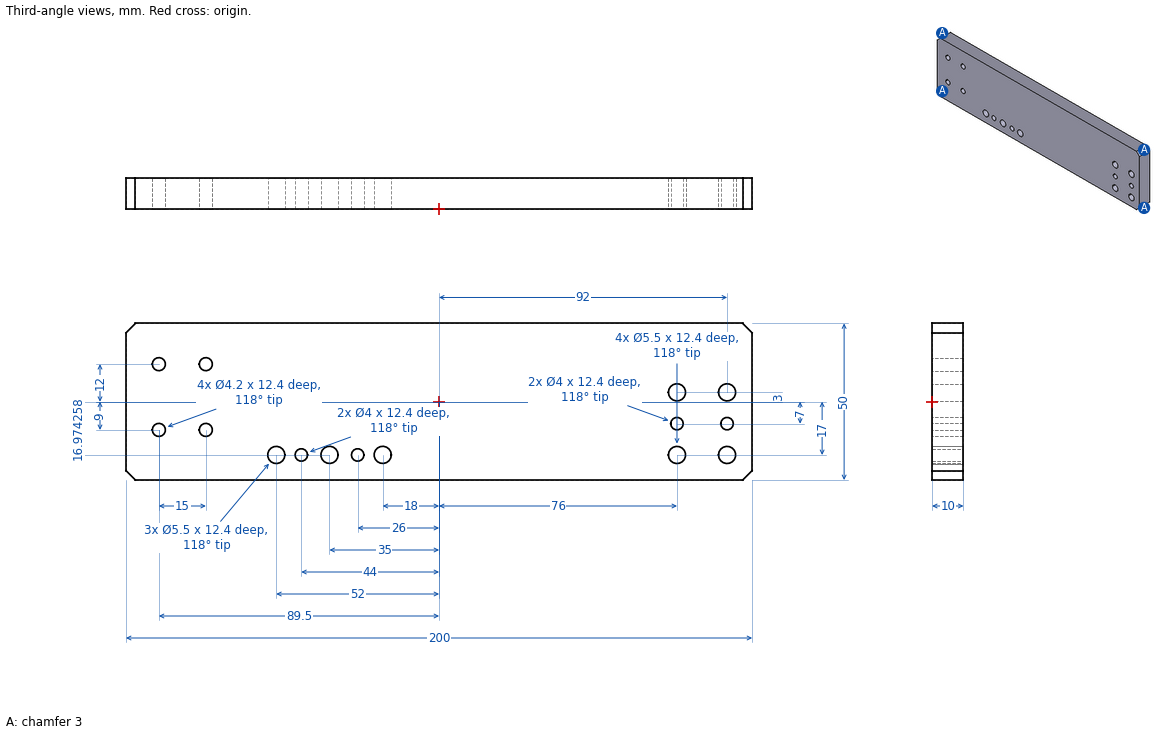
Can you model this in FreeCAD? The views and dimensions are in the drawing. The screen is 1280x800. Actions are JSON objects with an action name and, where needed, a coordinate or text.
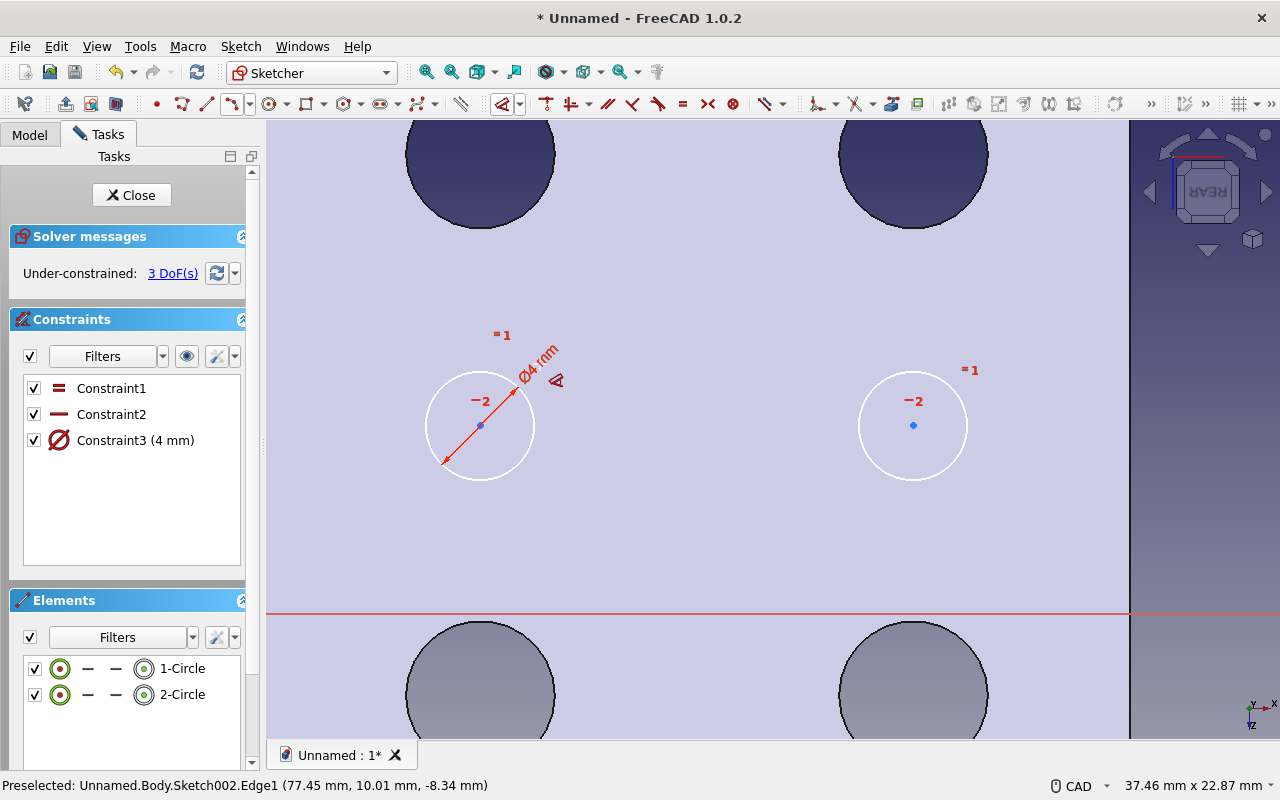
{"action": "left_click", "coordinate": [480, 426]}
{"action": "left_click", "coordinate": [514, 520]}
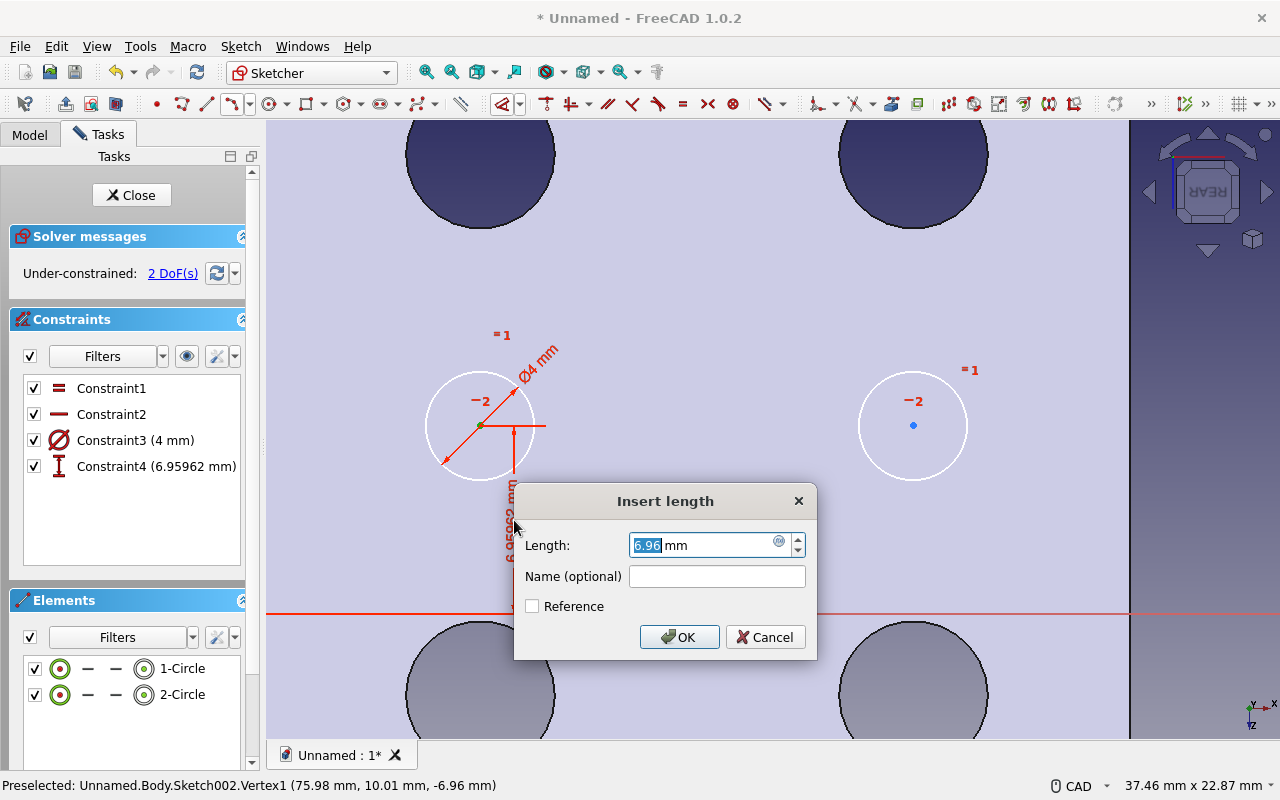
{"action": "type", "text": "7"}
{"action": "key", "text": "Return"}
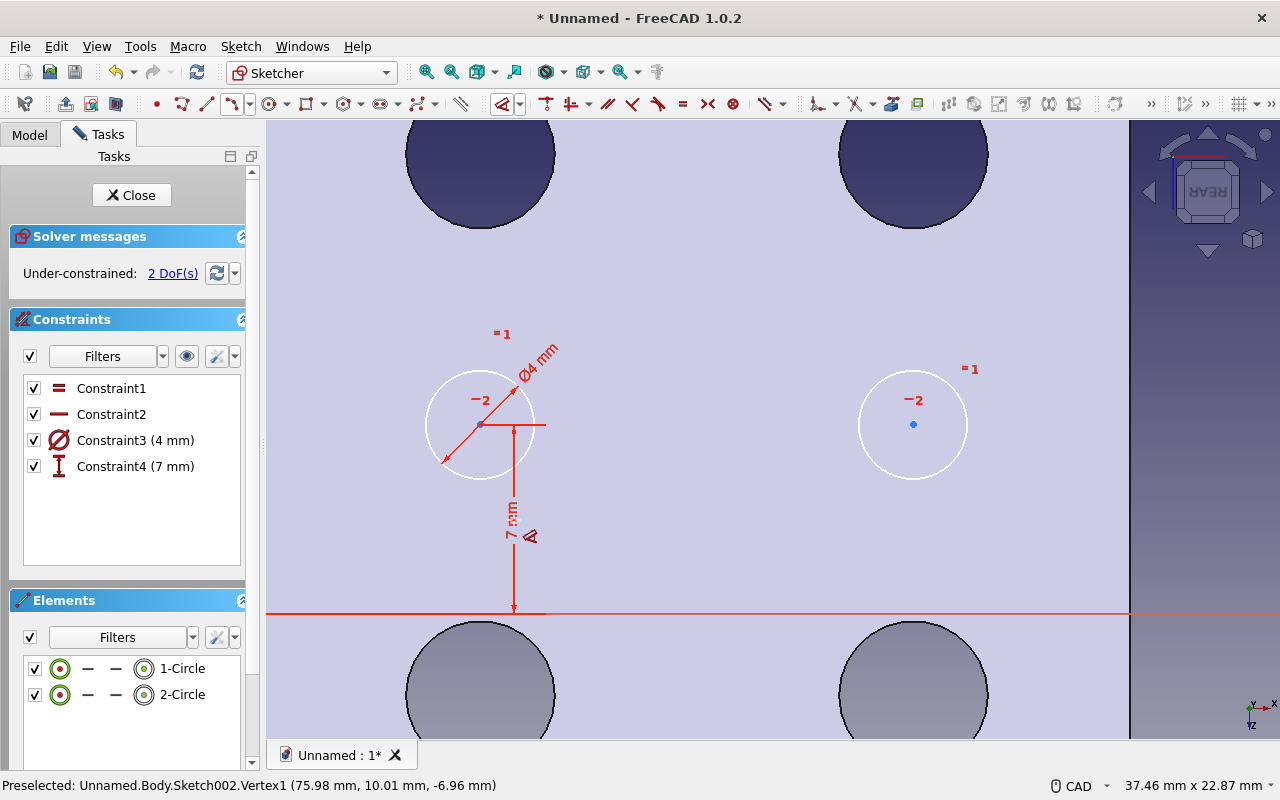
{"action": "left_click", "coordinate": [480, 425]}
{"action": "left_click", "coordinate": [387, 648]}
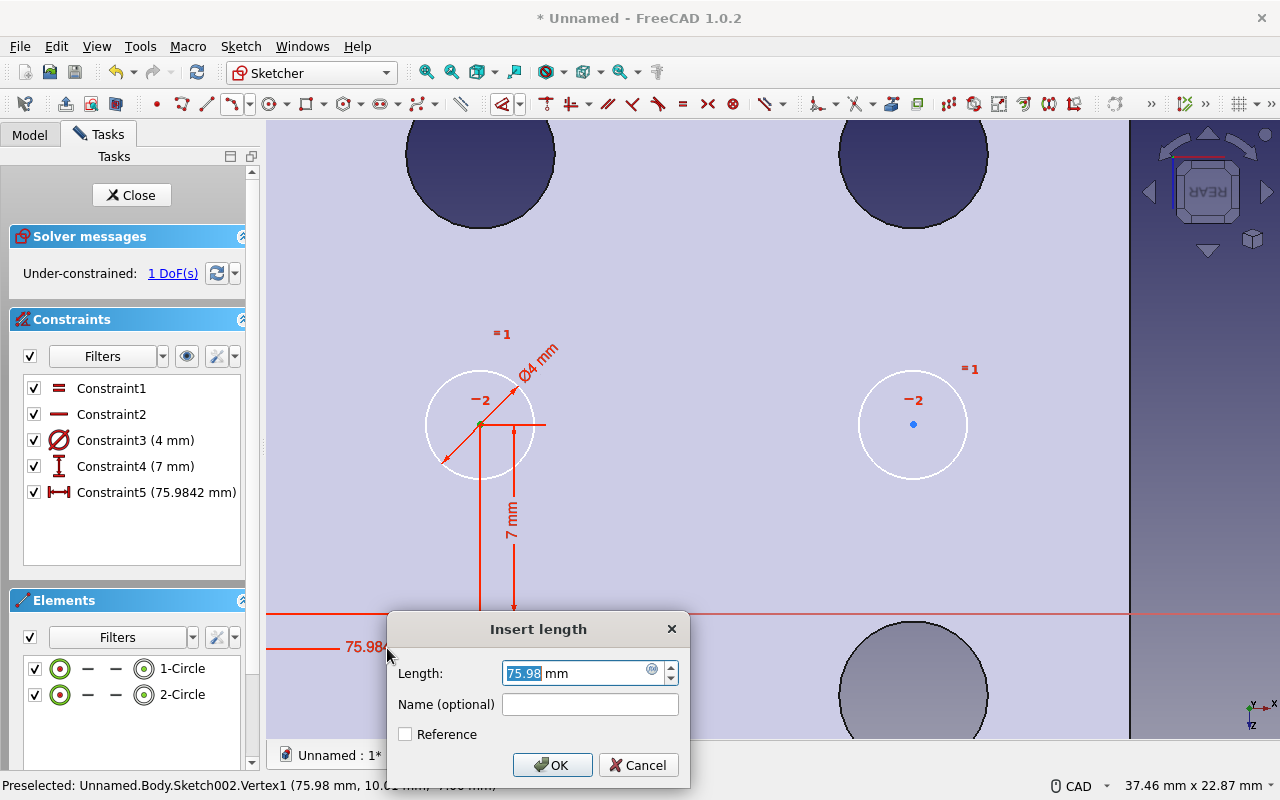
{"action": "type", "text": "76"}
{"action": "key", "text": "Return"}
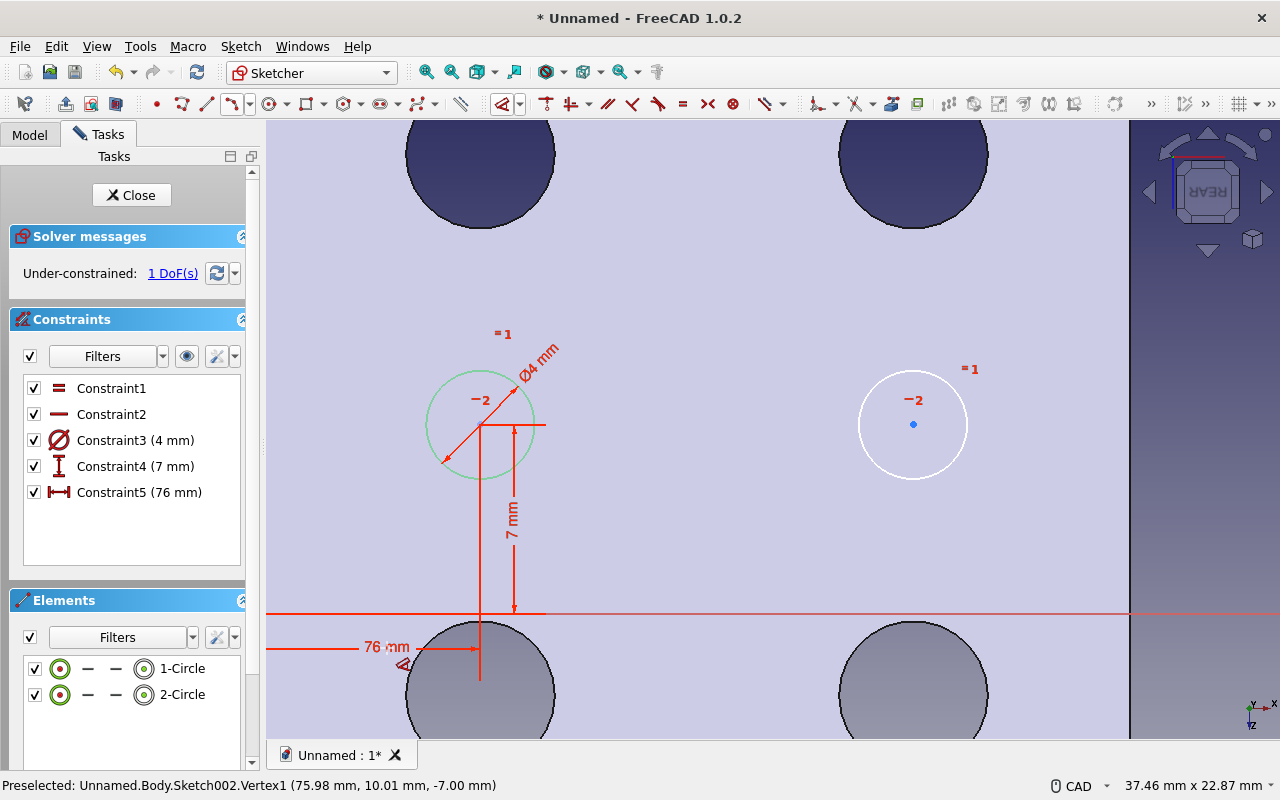
{"action": "left_click", "coordinate": [913, 425]}
{"action": "left_click", "coordinate": [604, 648]}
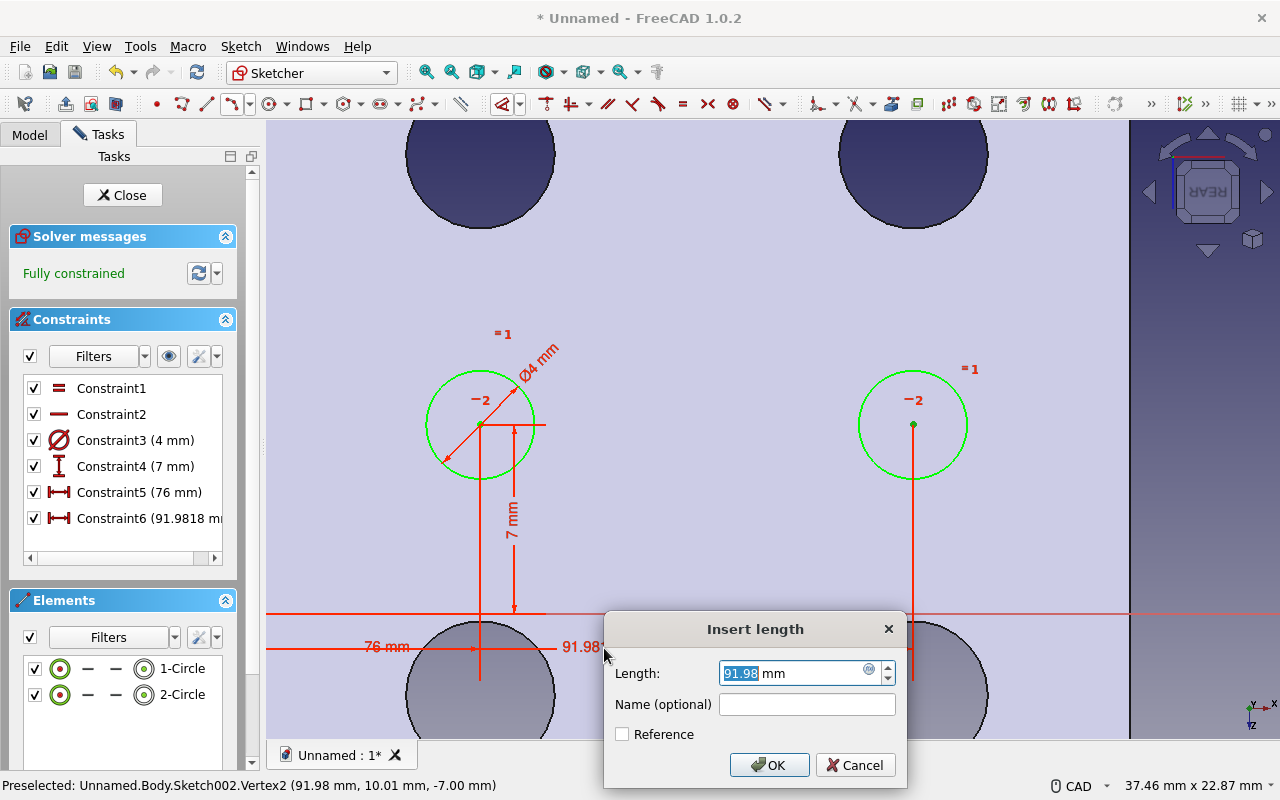
{"action": "type", "text": "92"}
{"action": "key", "text": "Return"}
{"action": "key", "text": "Escape"}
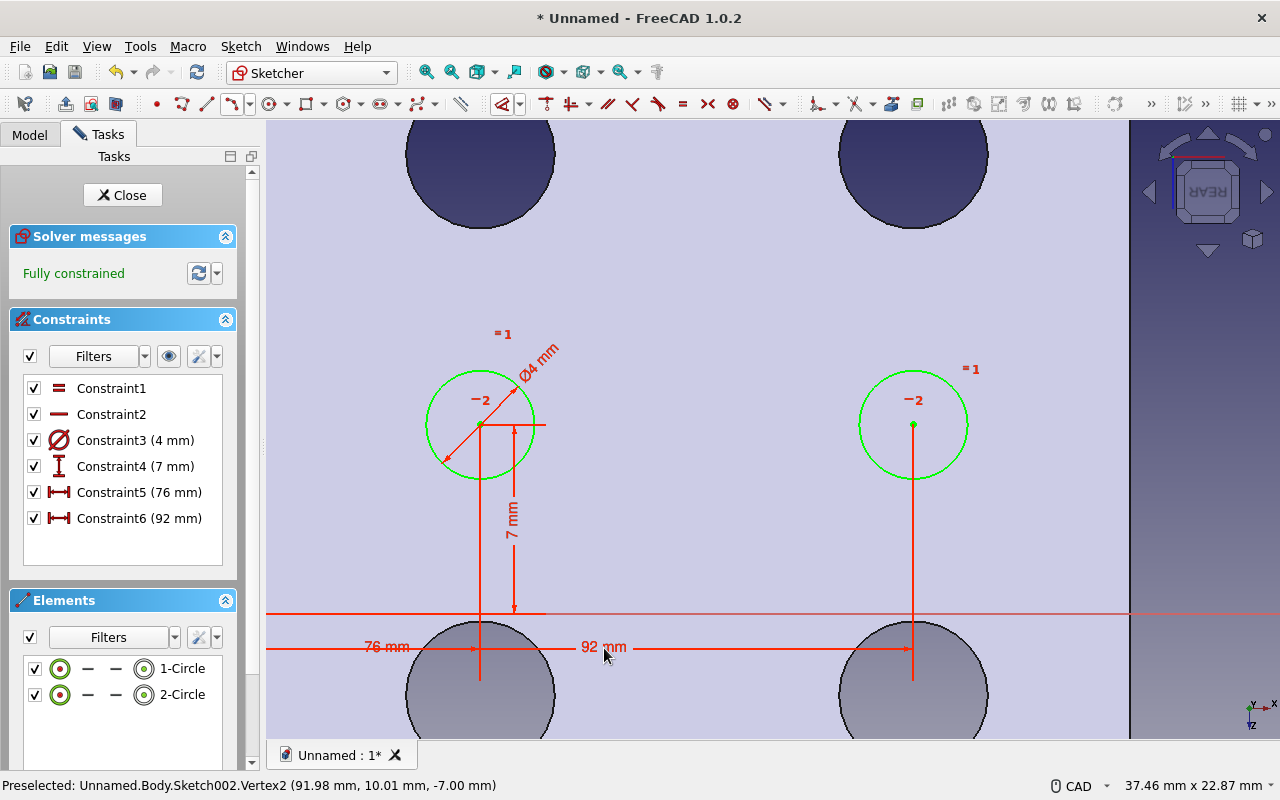
{"action": "left_click", "coordinate": [123, 195]}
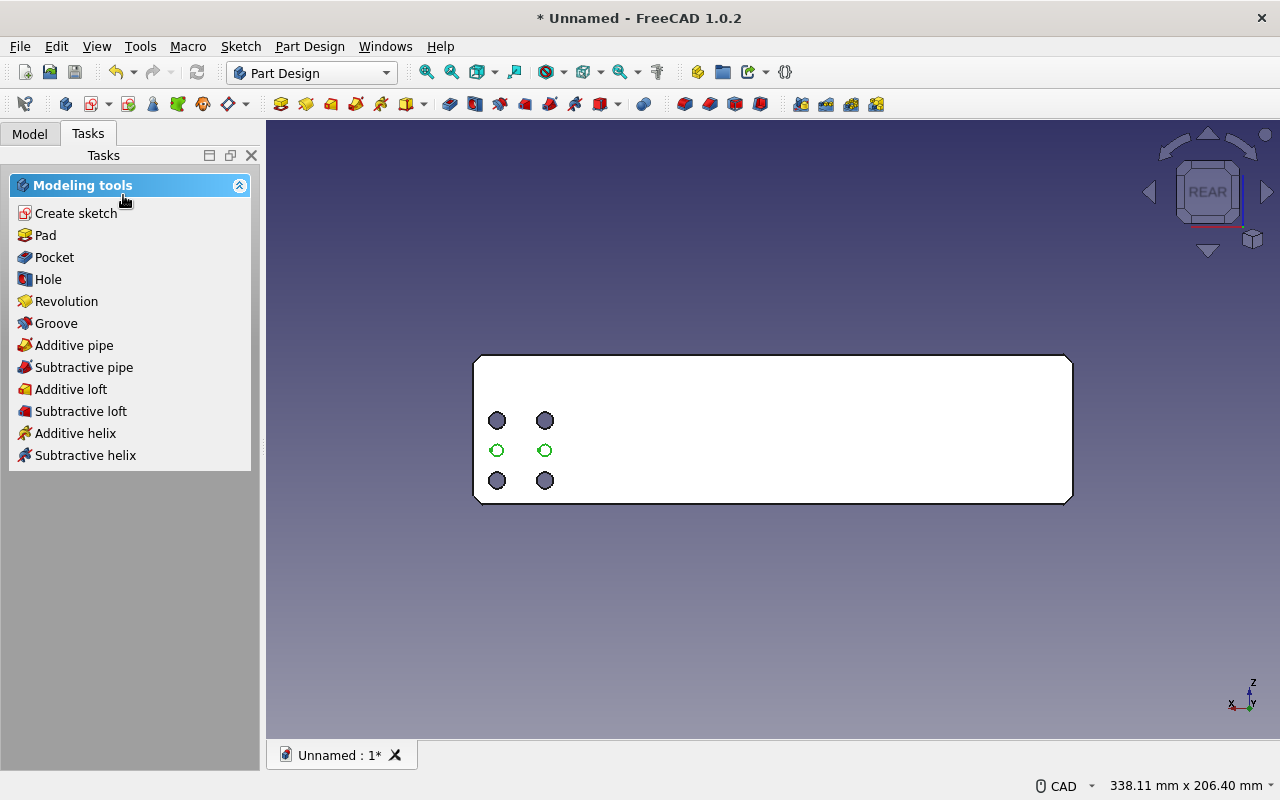
{"action": "left_click", "coordinate": [475, 104]}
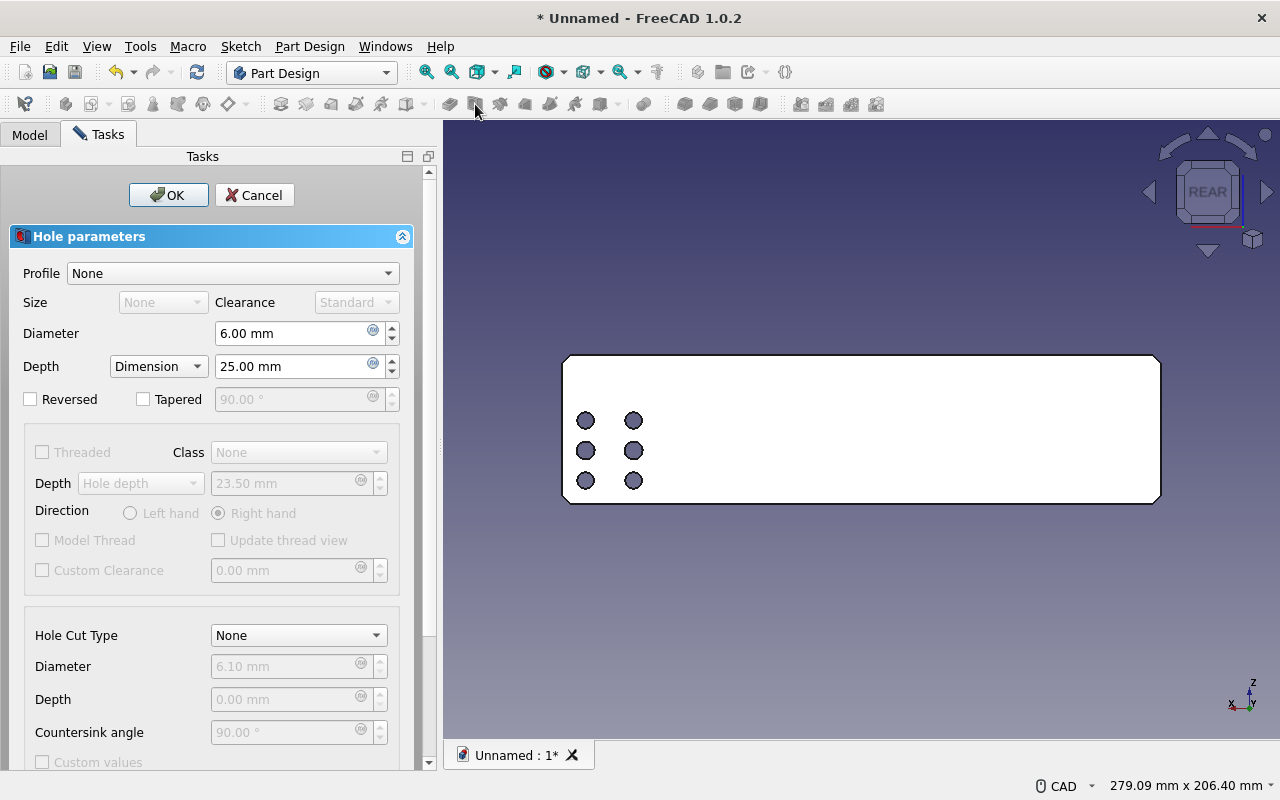
{"action": "triple_click", "coordinate": [300, 334]}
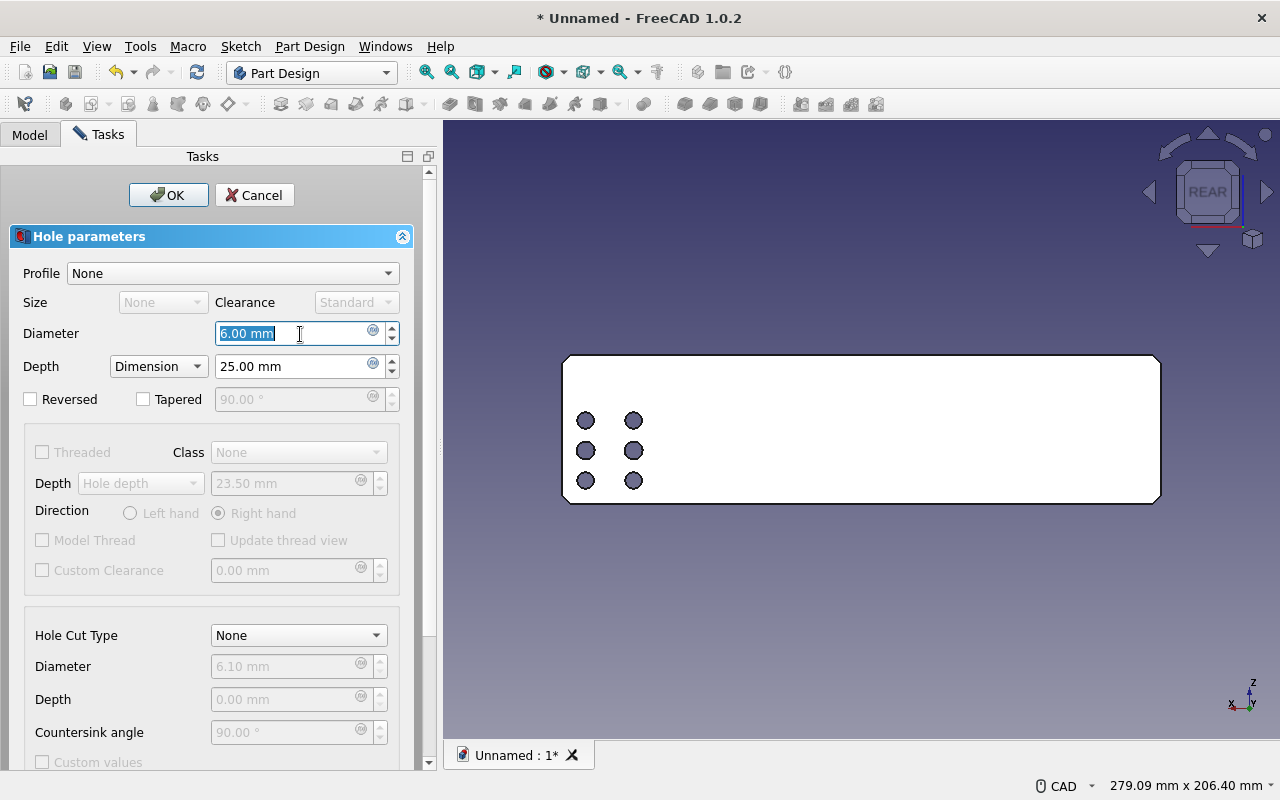
{"action": "type", "text": "4"}
{"action": "key", "text": "Tab"}